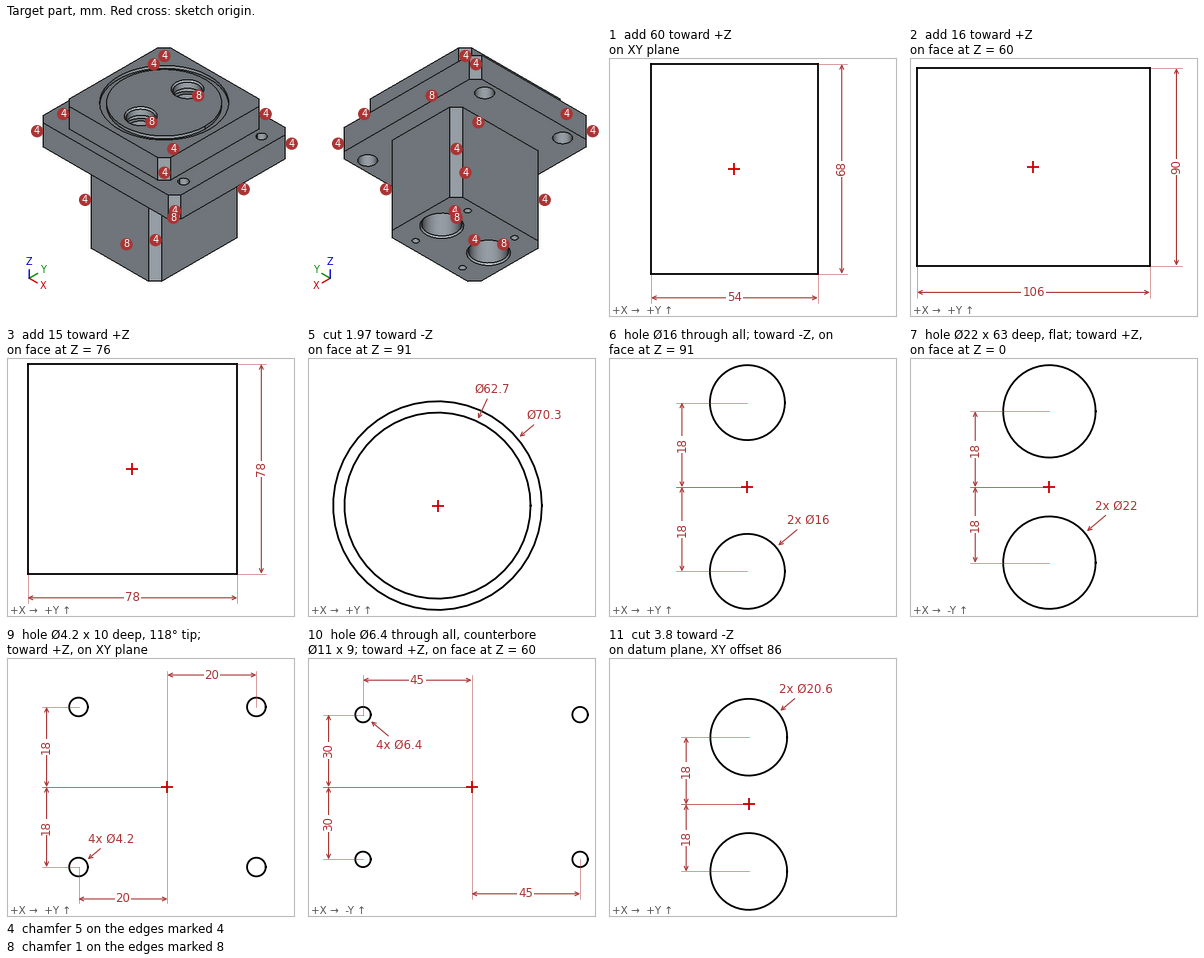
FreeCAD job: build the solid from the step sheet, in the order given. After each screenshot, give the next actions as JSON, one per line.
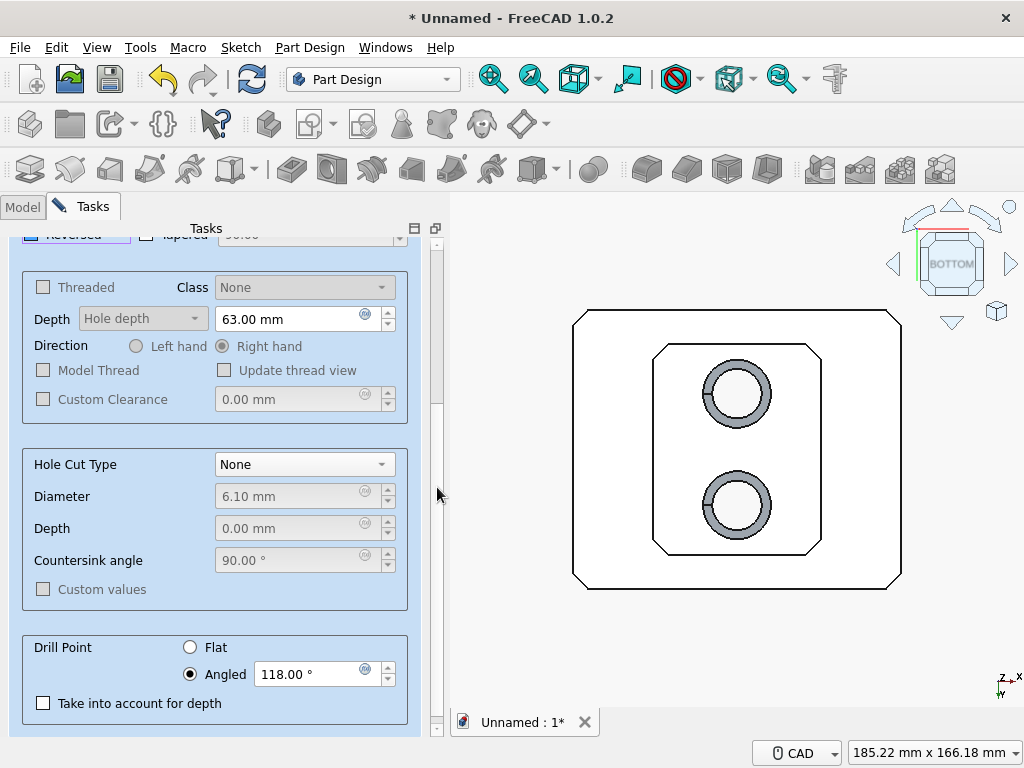
{"action": "left_click", "coordinate": [191, 647]}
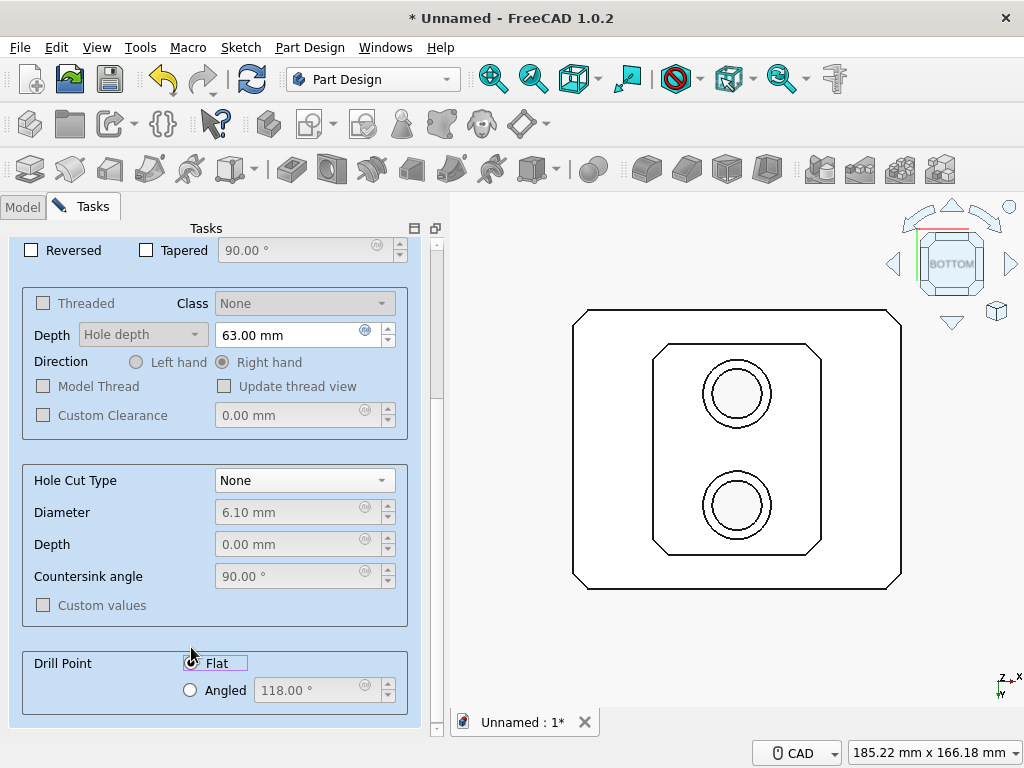
{"action": "scroll", "coordinate": [437, 487], "scroll_direction": "up", "scroll_amount": 5}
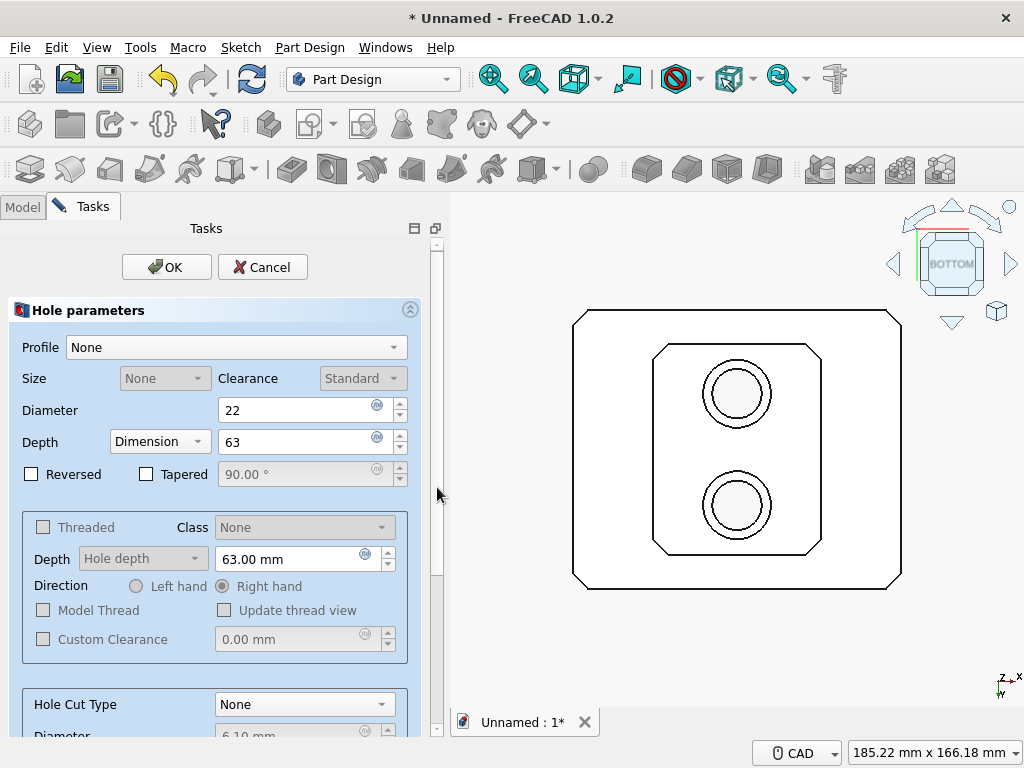
{"action": "left_click", "coordinate": [167, 267]}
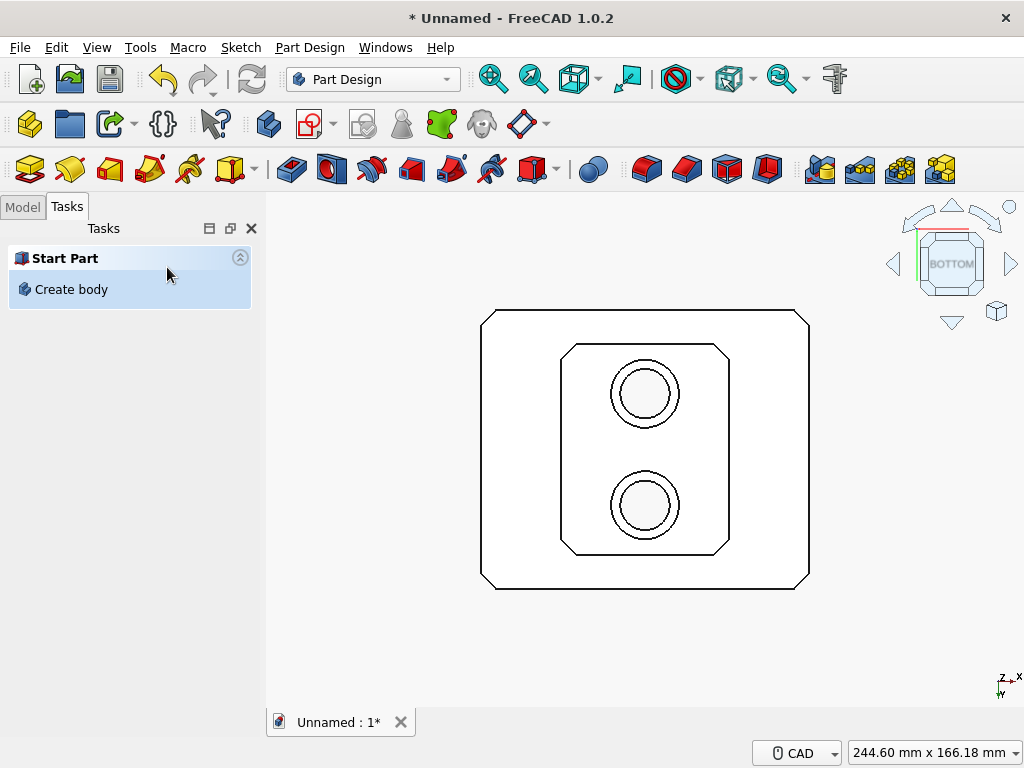
{"action": "left_click", "coordinate": [673, 413]}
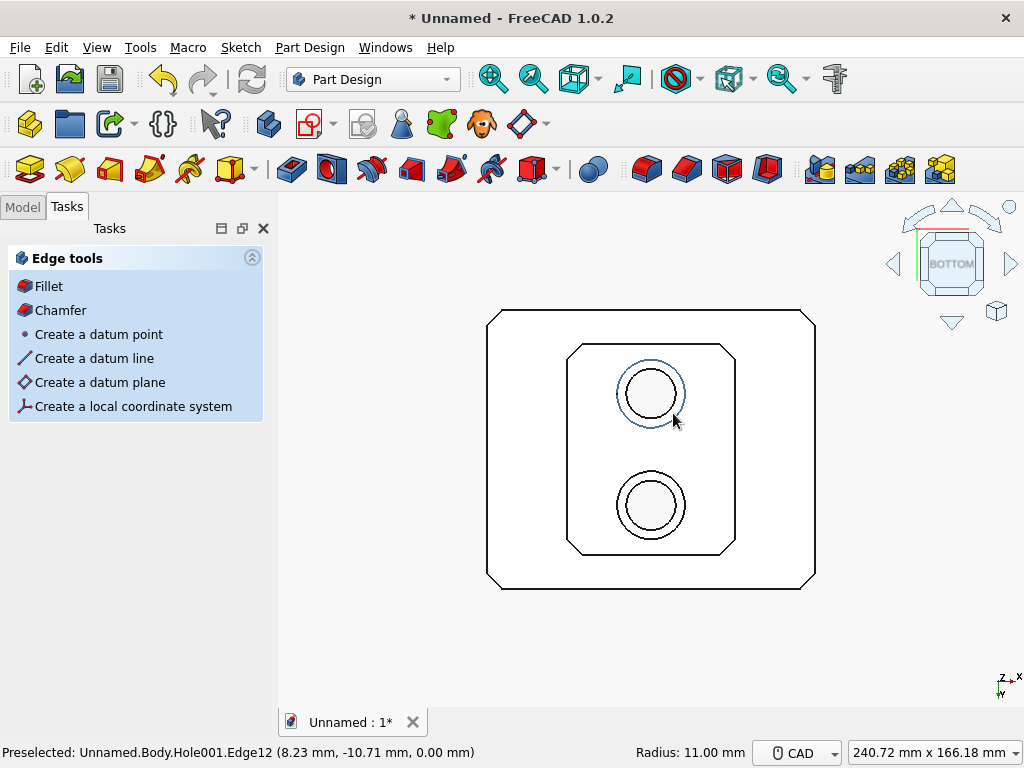
{"action": "left_click", "coordinate": [679, 484], "text": "ctrl"}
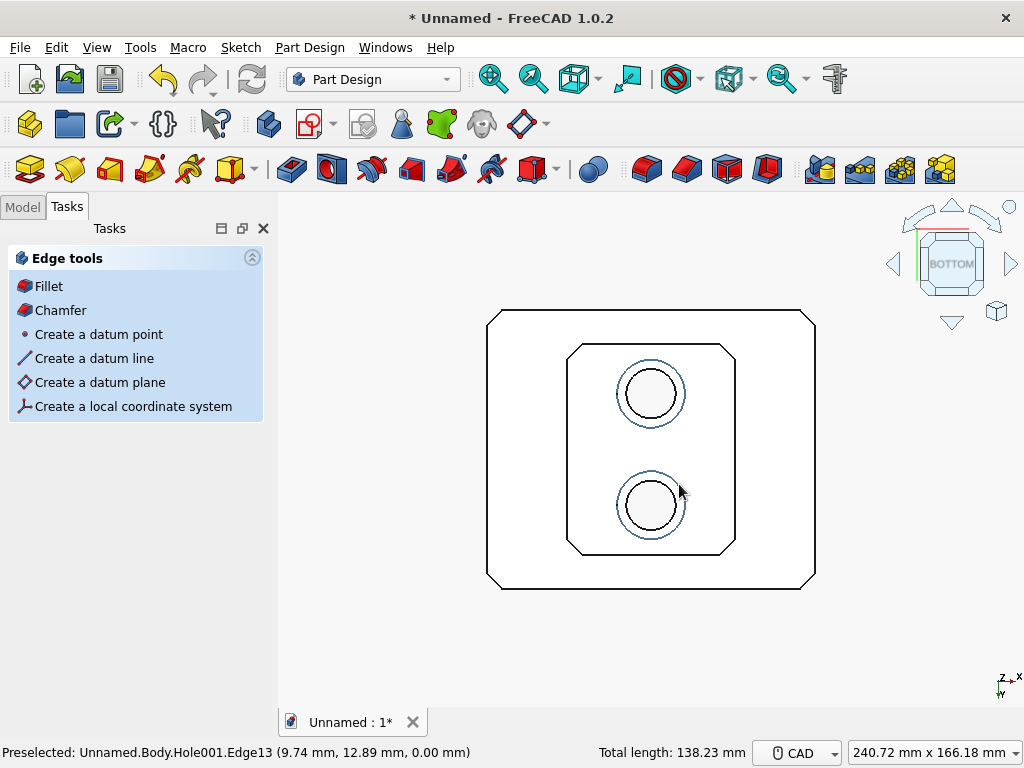
{"action": "key", "text": "0"}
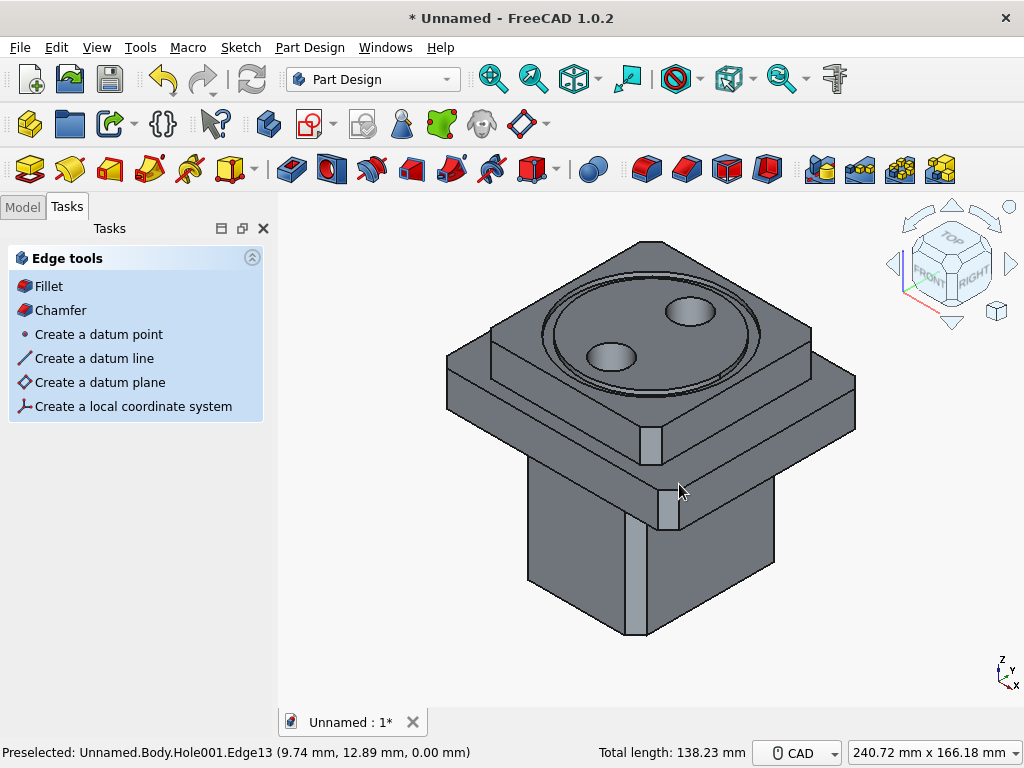
{"action": "left_click", "coordinate": [673, 300], "text": "ctrl"}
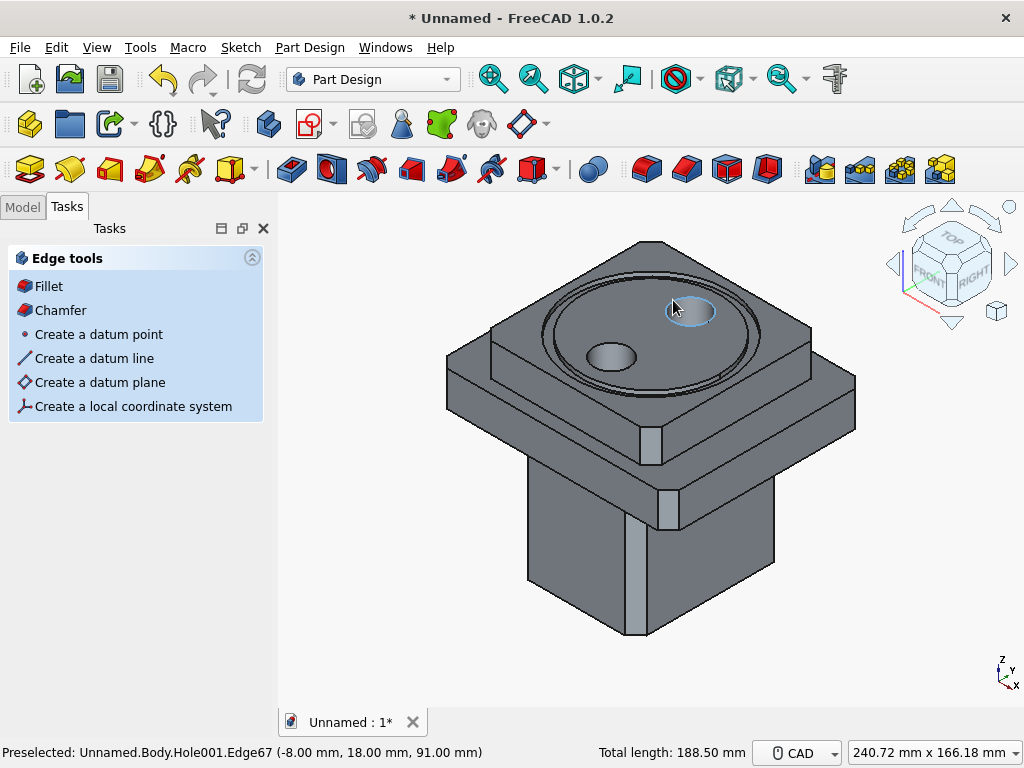
{"action": "left_click", "coordinate": [594, 346], "text": "ctrl"}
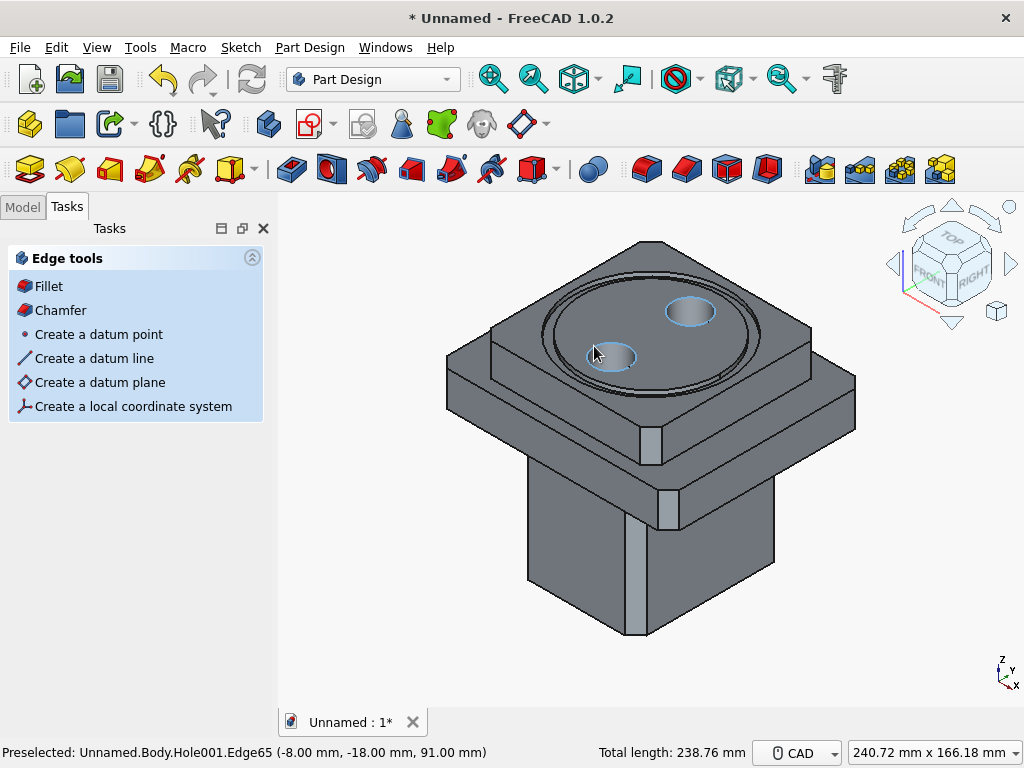
{"action": "left_click", "coordinate": [688, 170]}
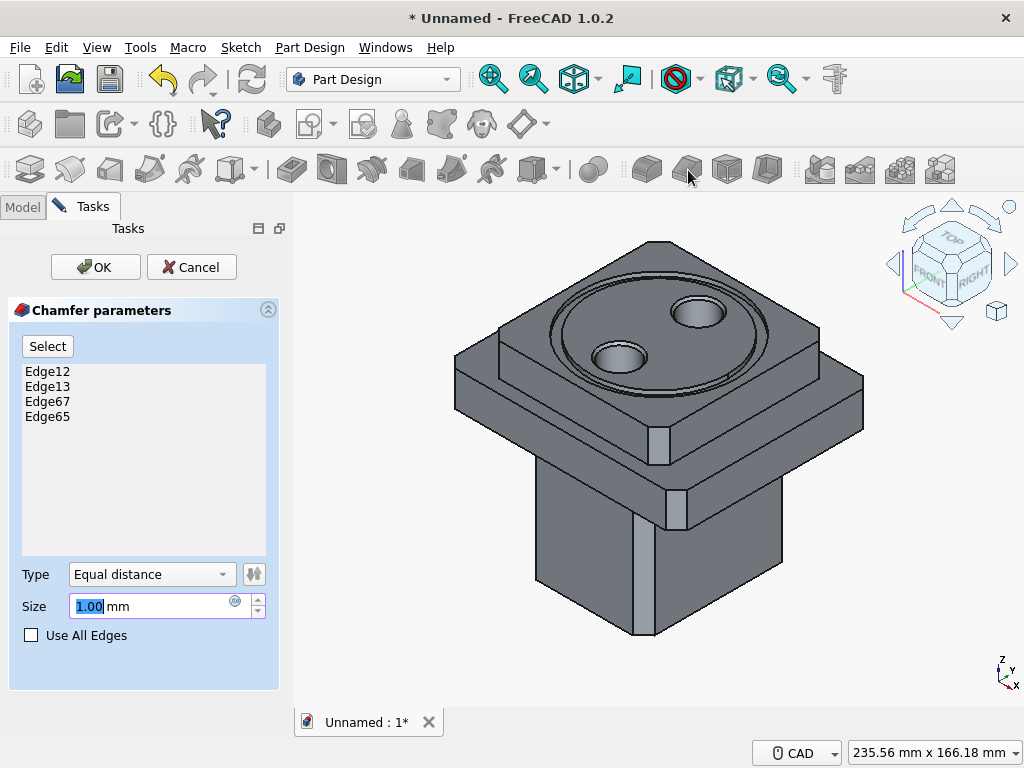
{"action": "type", "text": "1"}
{"action": "key", "text": "Tab"}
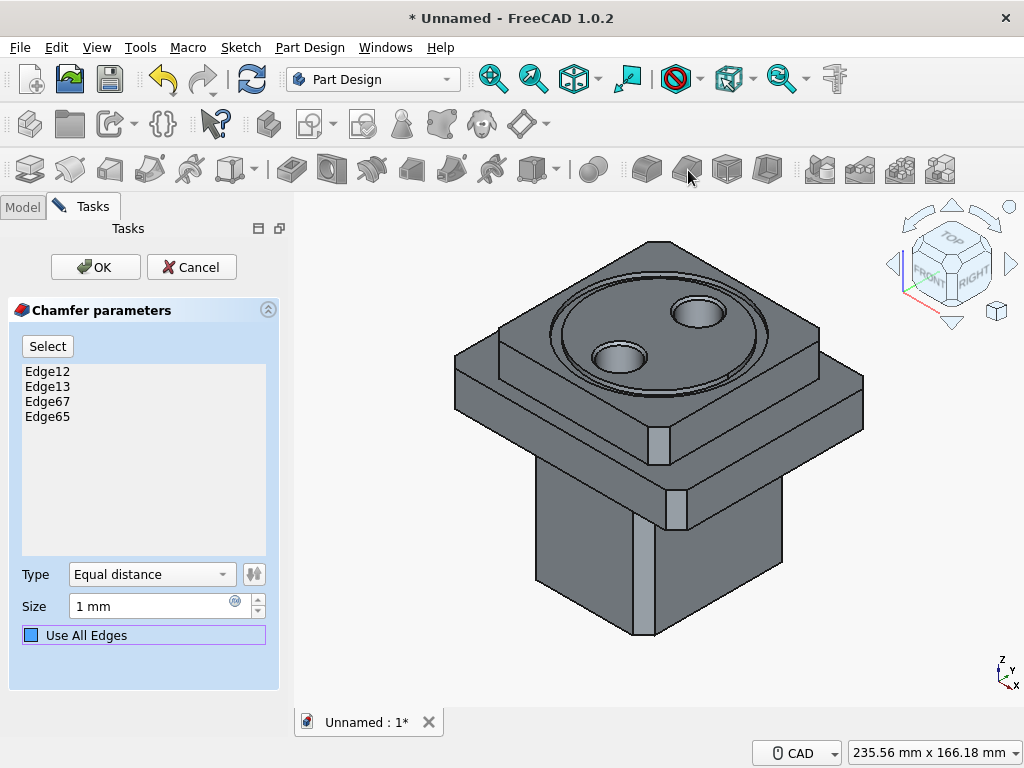
{"action": "left_click", "coordinate": [96, 267]}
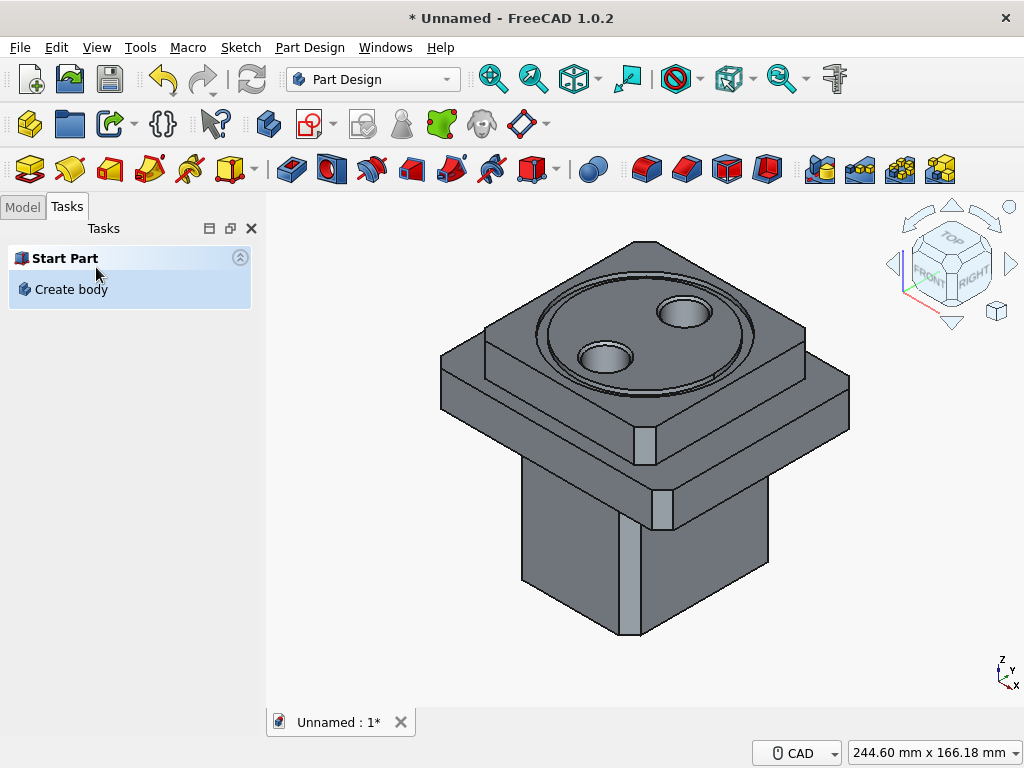
{"action": "left_click", "coordinate": [310, 124]}